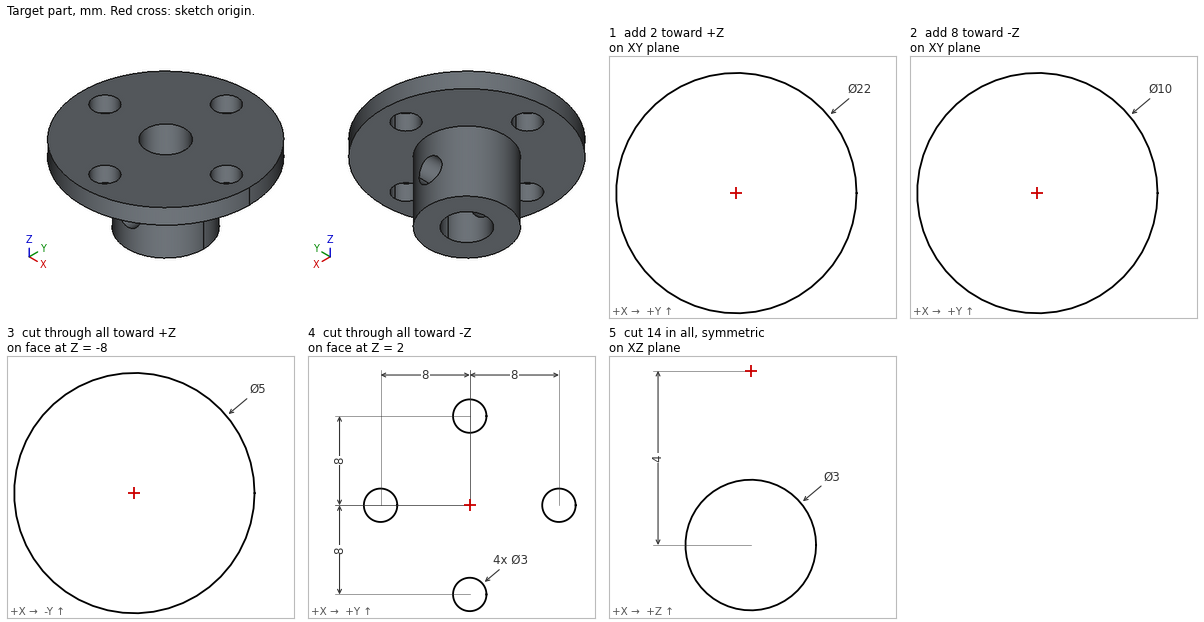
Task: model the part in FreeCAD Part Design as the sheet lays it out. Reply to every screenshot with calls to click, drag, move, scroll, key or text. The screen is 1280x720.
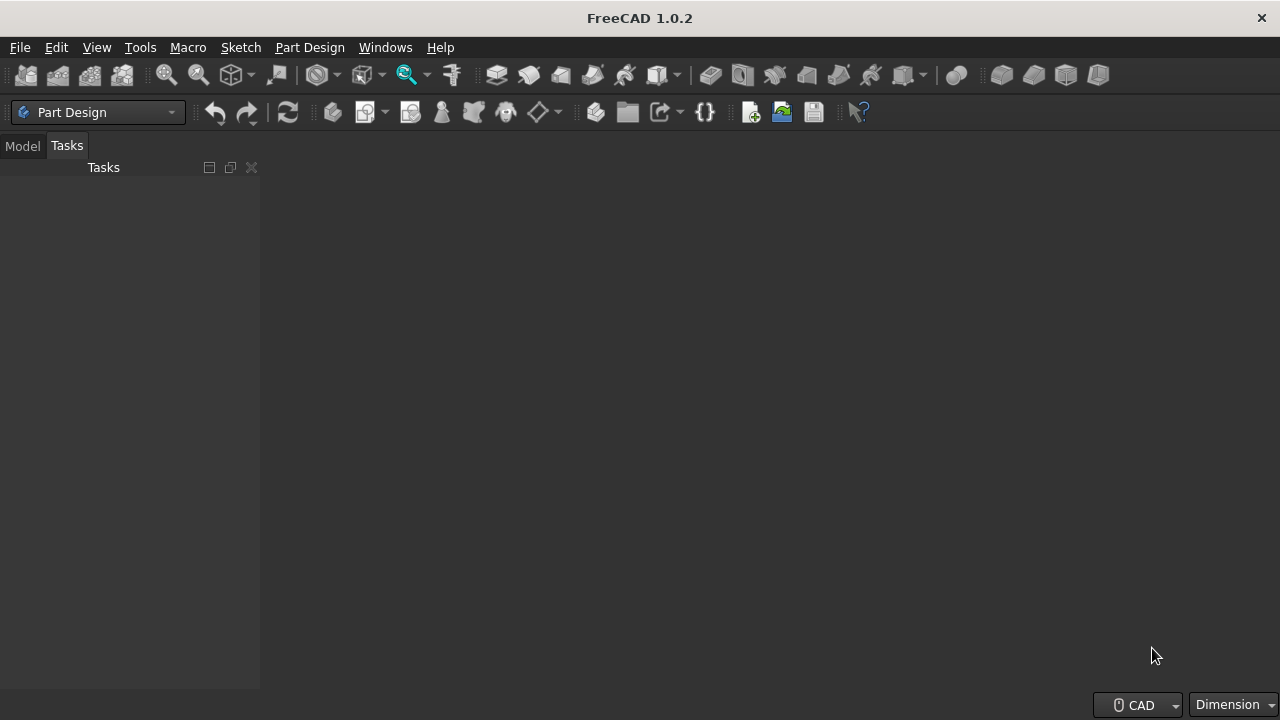
key(ctrl+n)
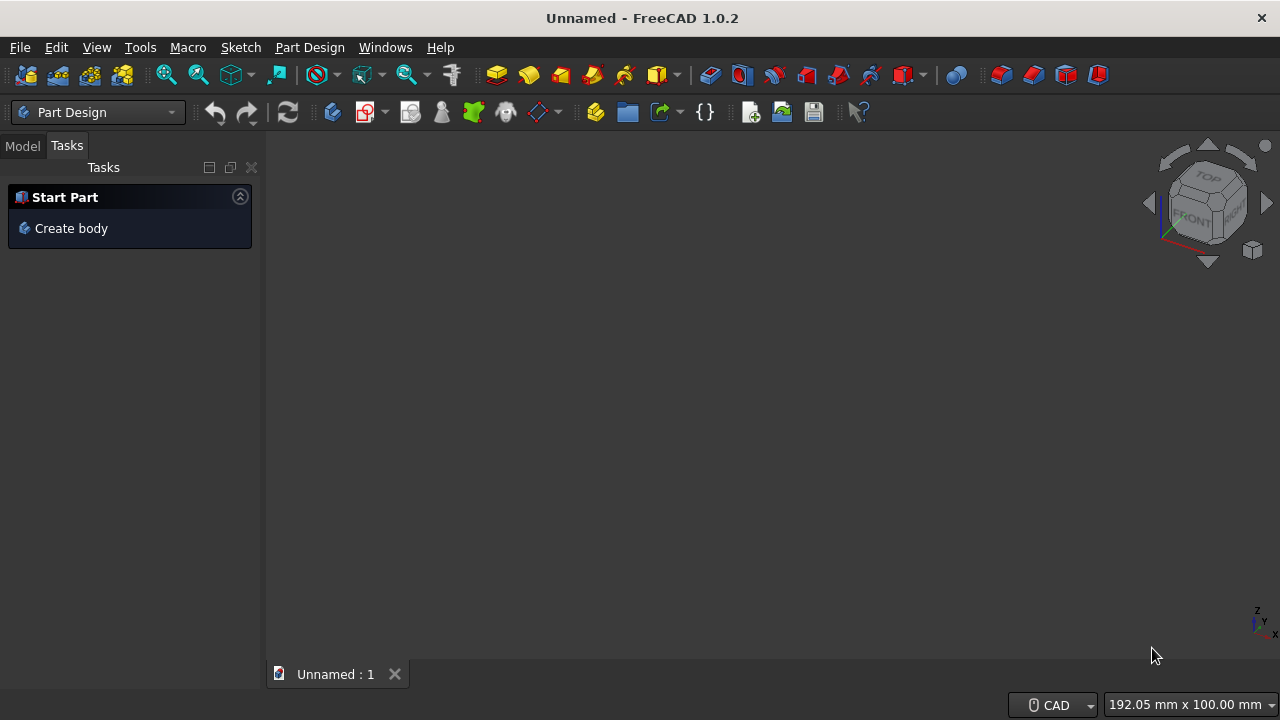
click(366, 112)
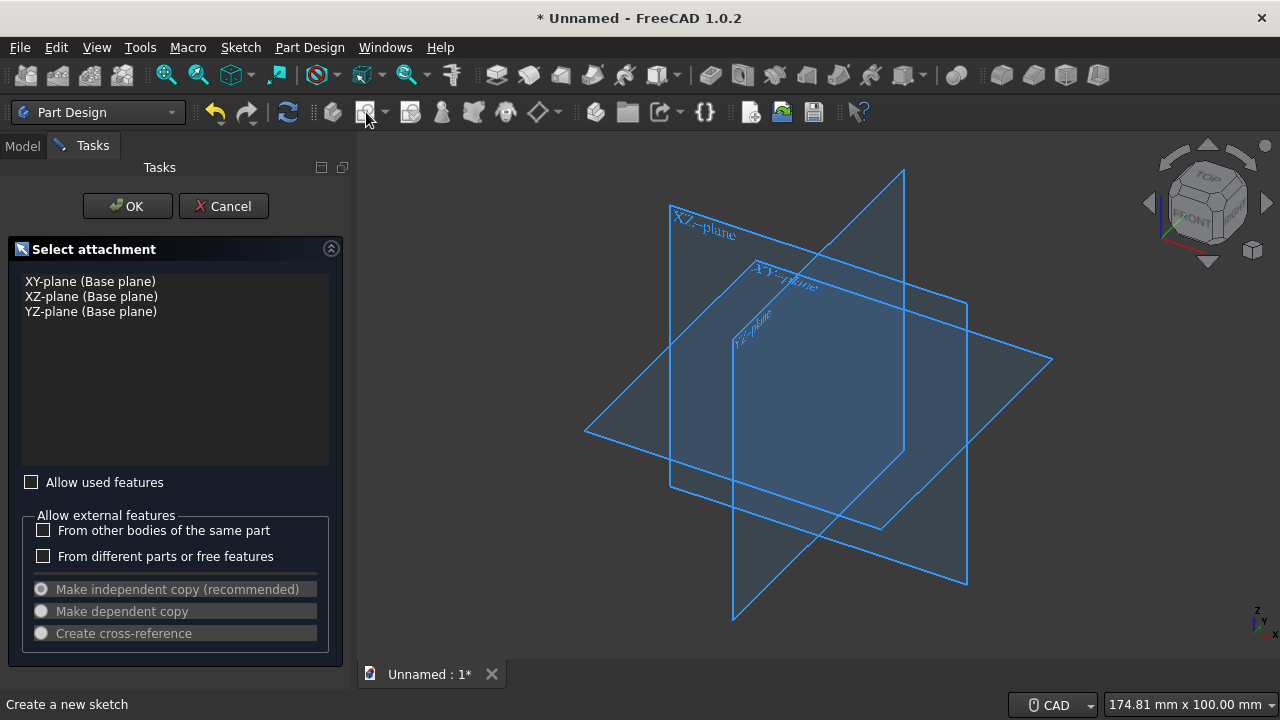
click(82, 282)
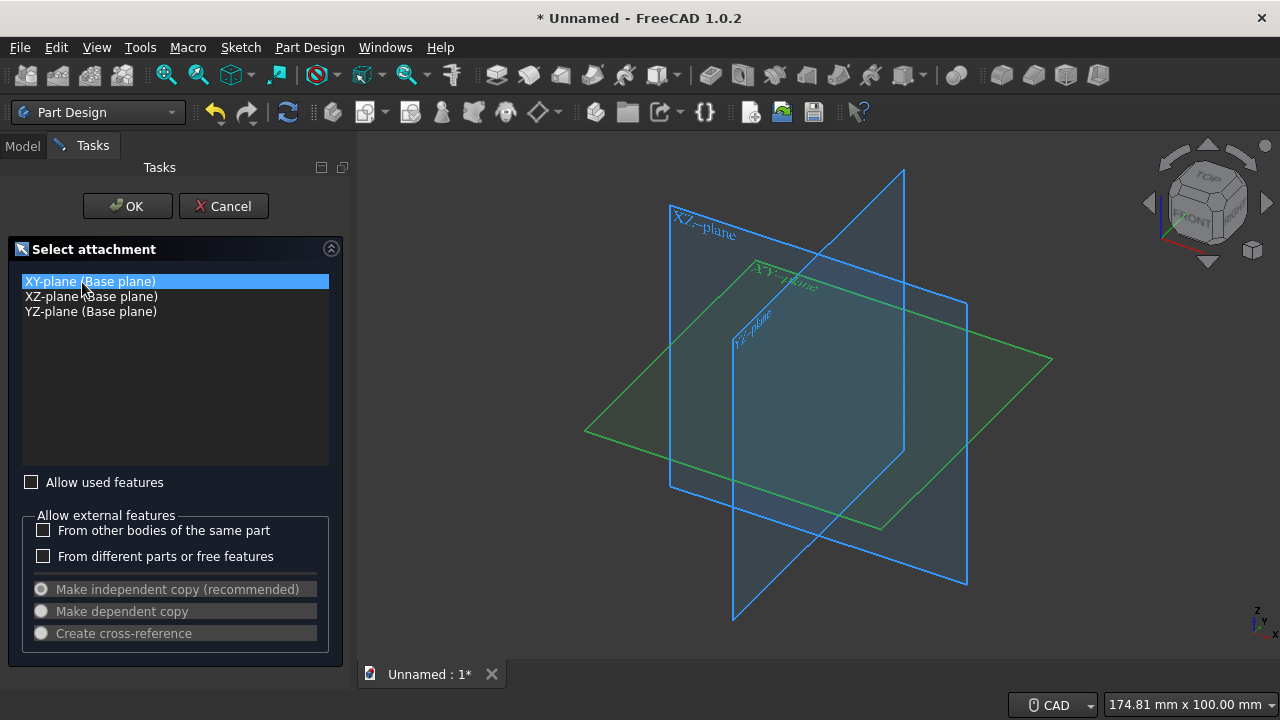
click(128, 206)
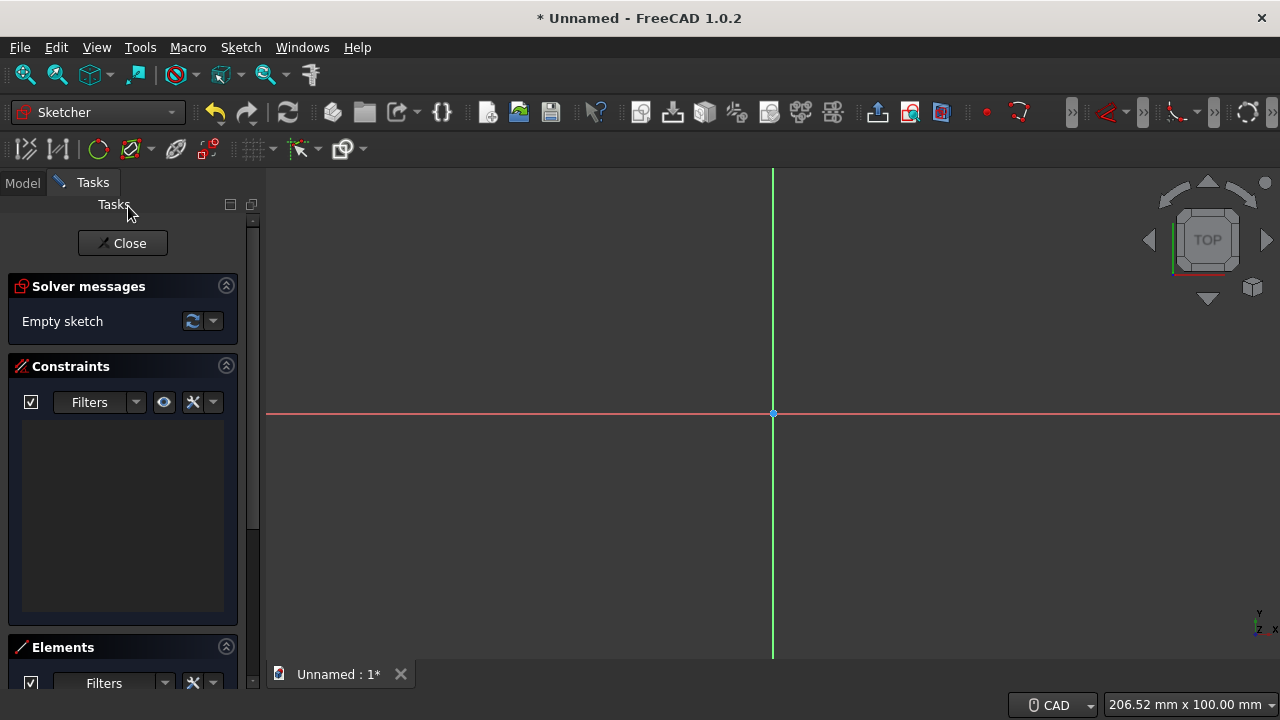
scroll(813, 414, up, 5)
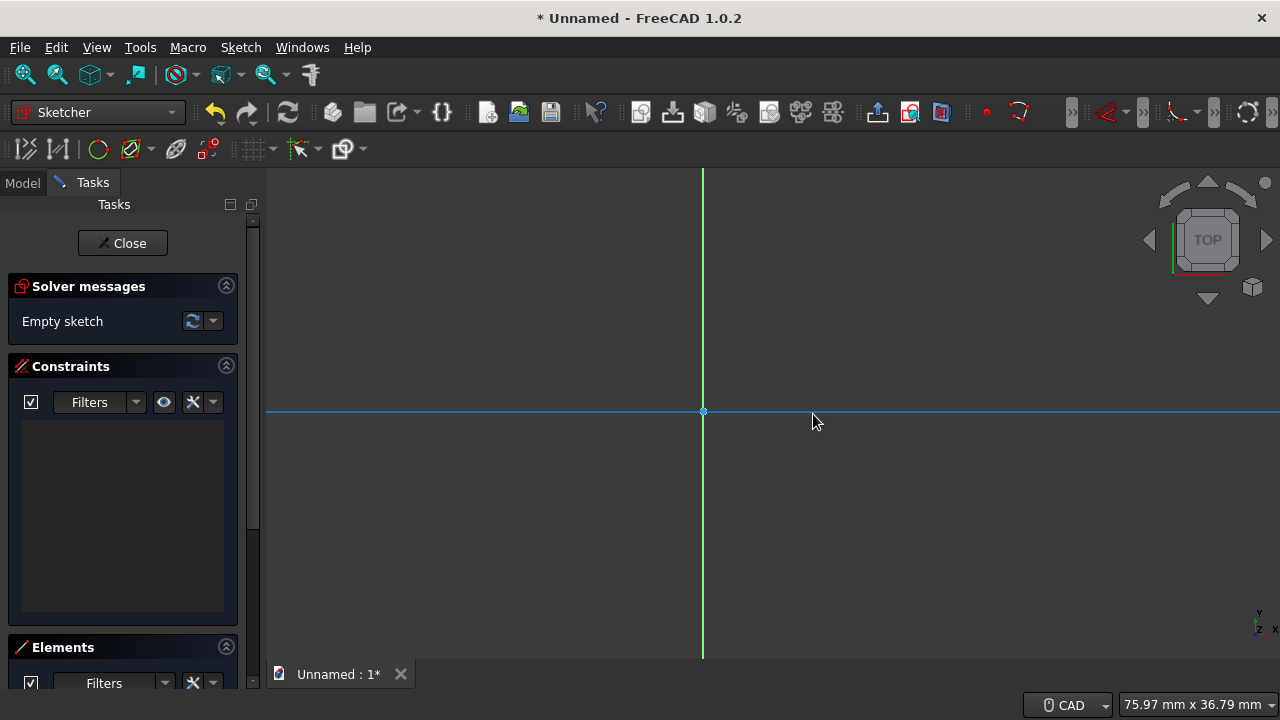
key(g)
key(c)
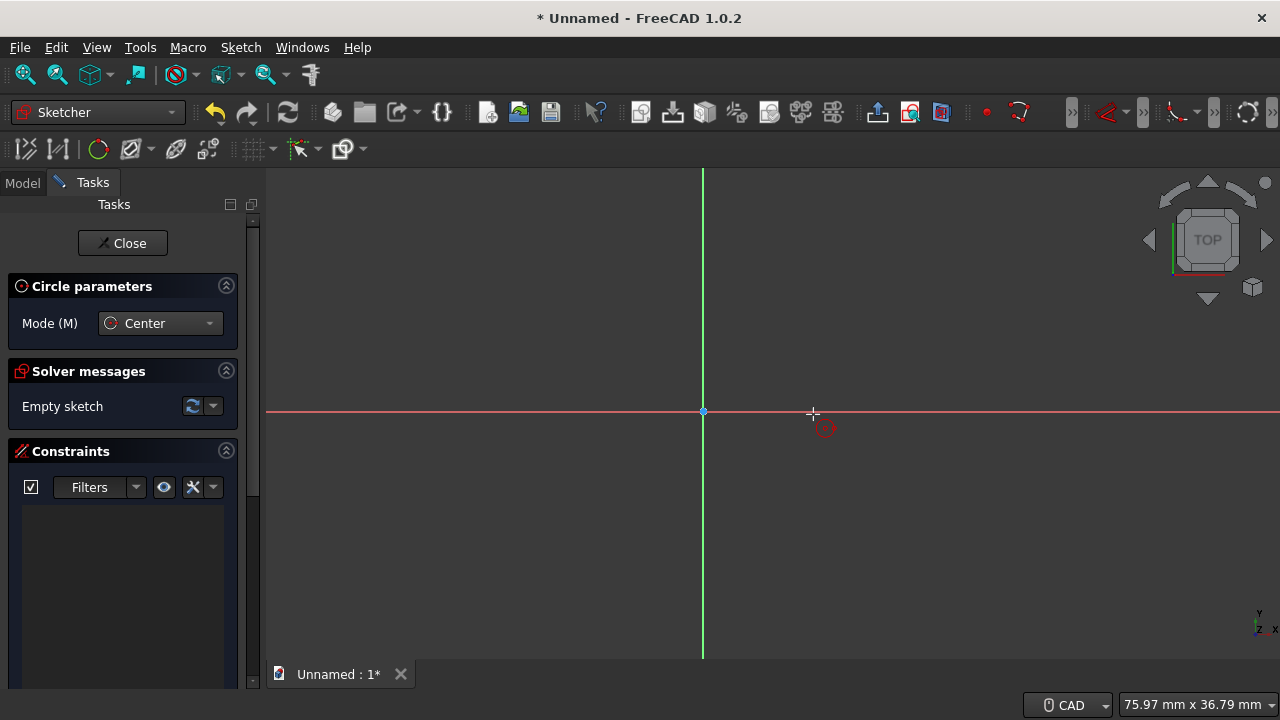
click(703, 412)
click(807, 308)
key(Escape)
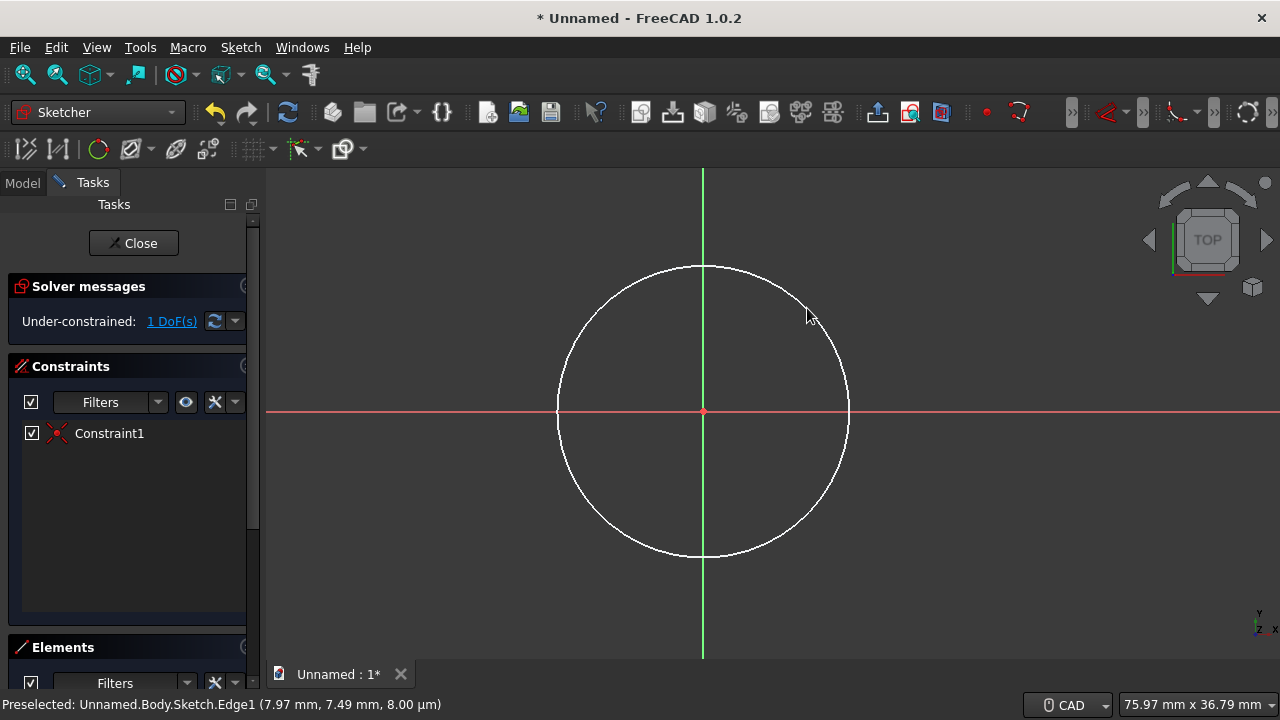
click(806, 308)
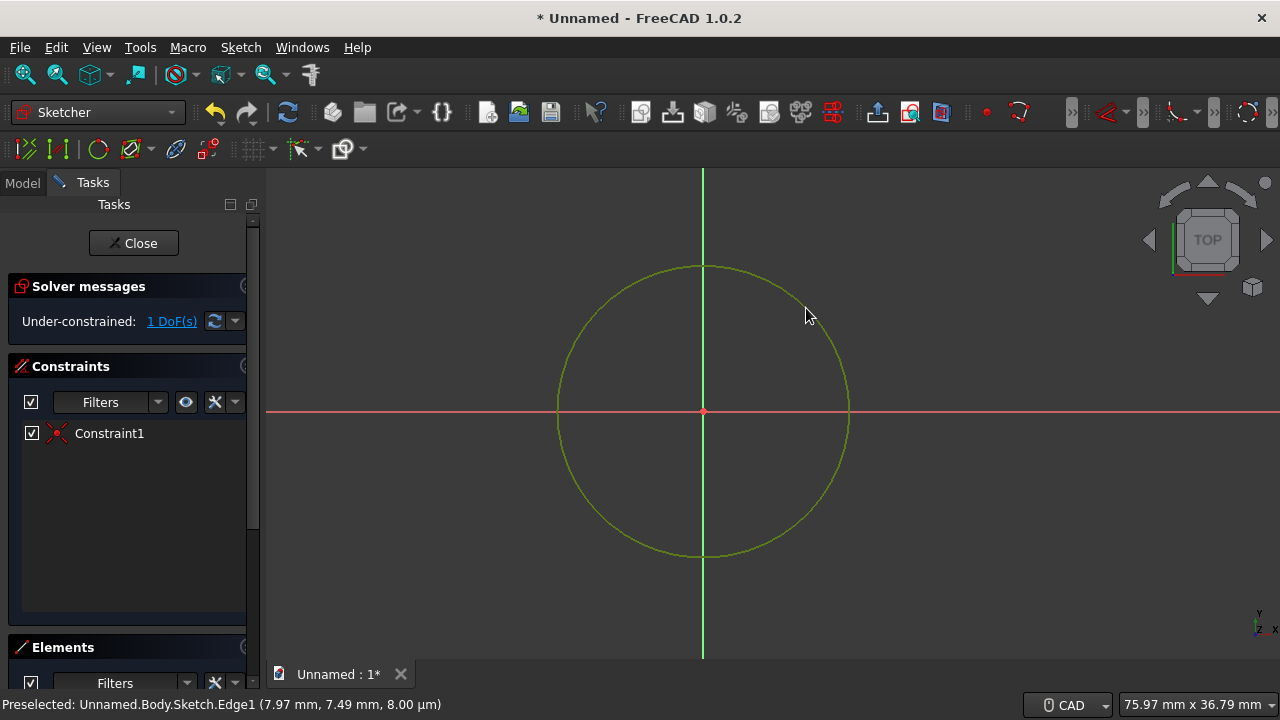
key(k)
key(o)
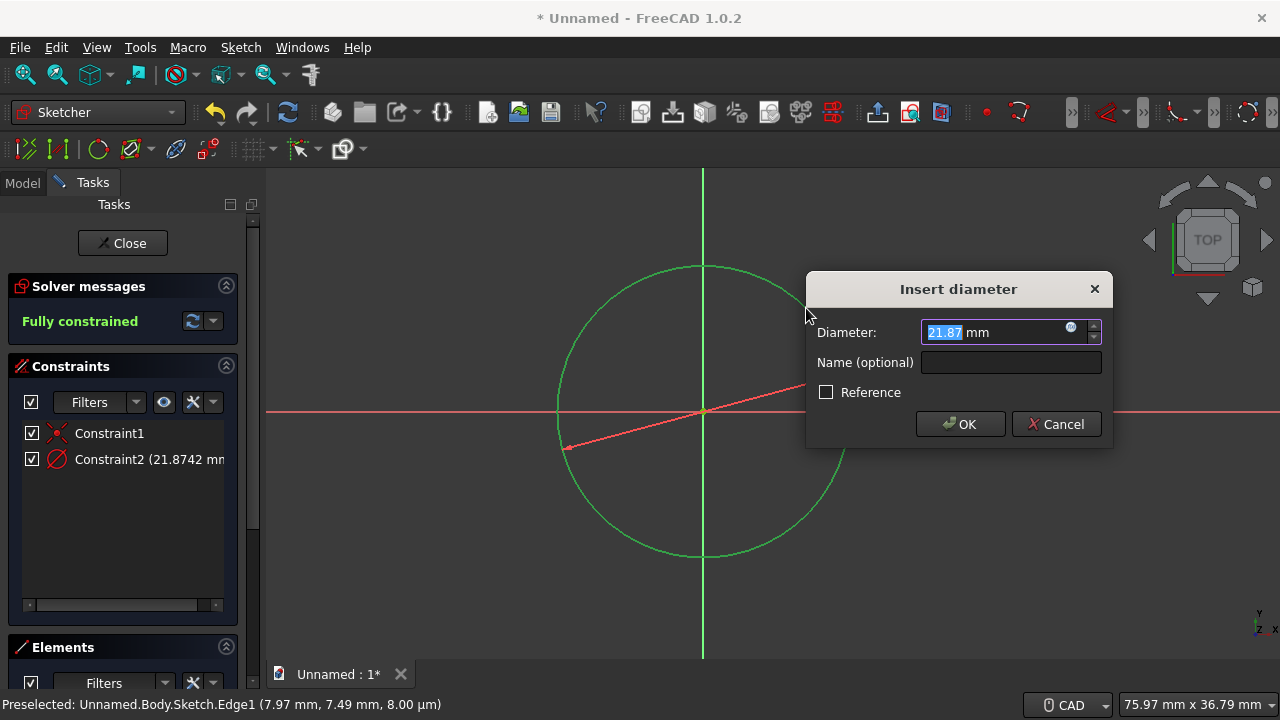
text(22)
key(Return)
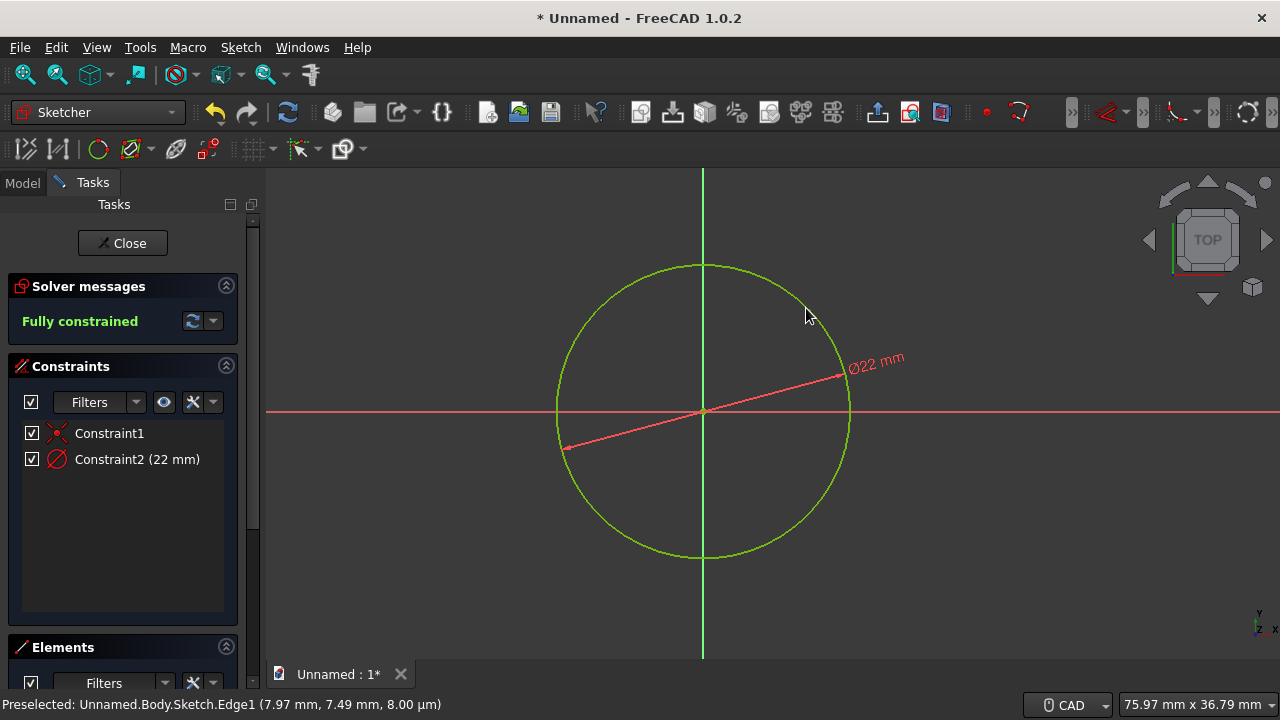
click(123, 243)